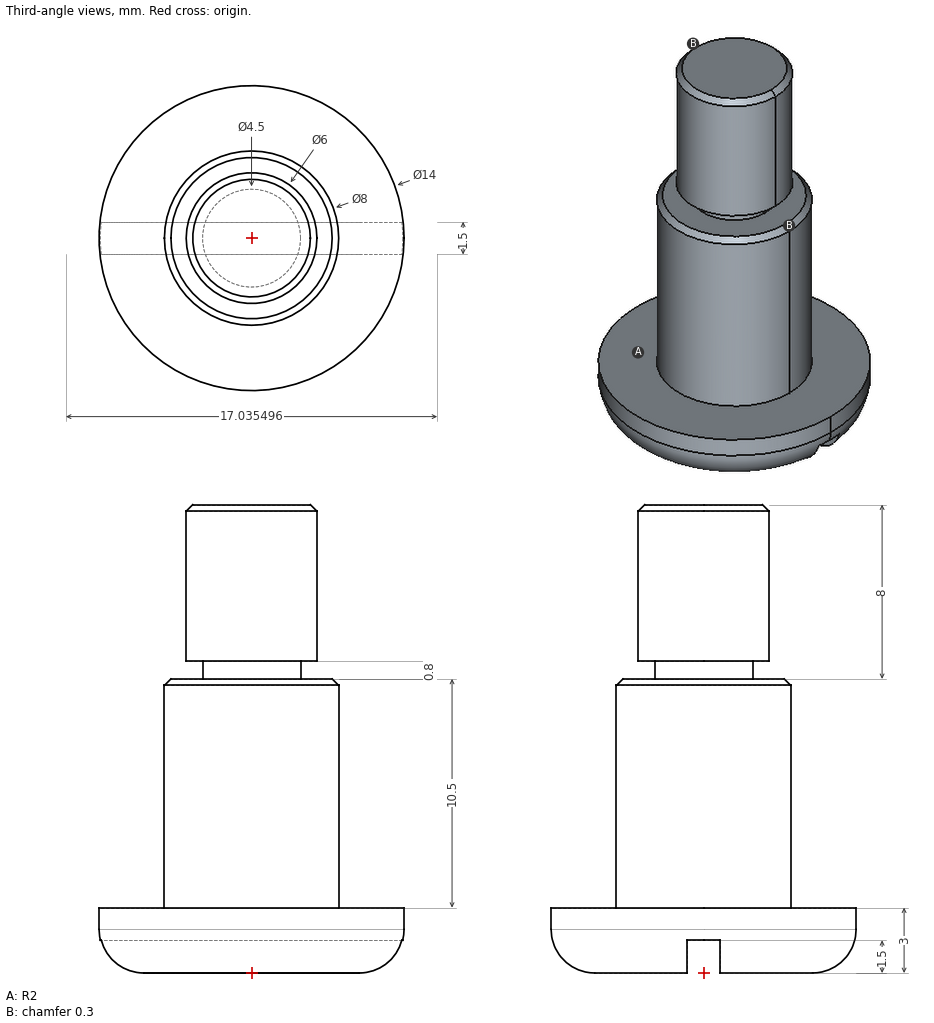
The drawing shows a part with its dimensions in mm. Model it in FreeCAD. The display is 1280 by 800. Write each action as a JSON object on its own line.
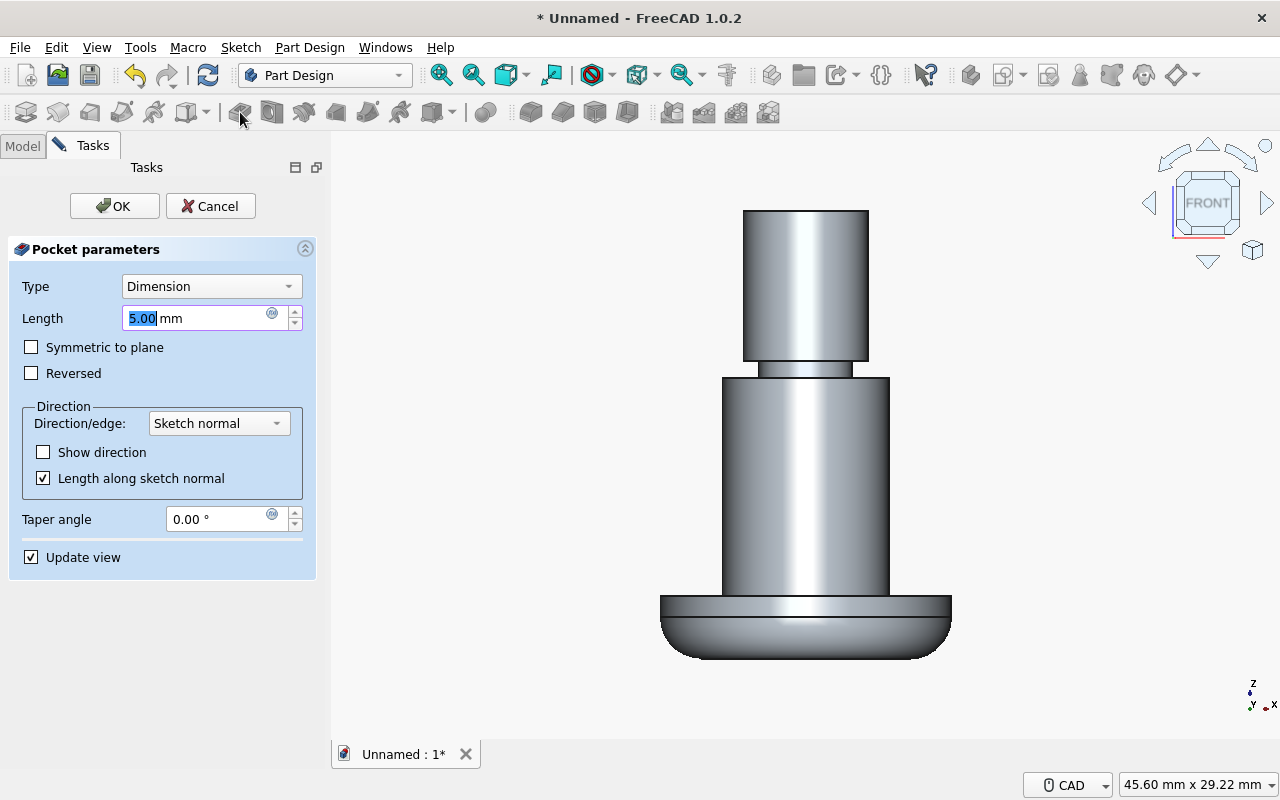
{"action": "type", "text": "1.5"}
{"action": "key", "text": "Tab"}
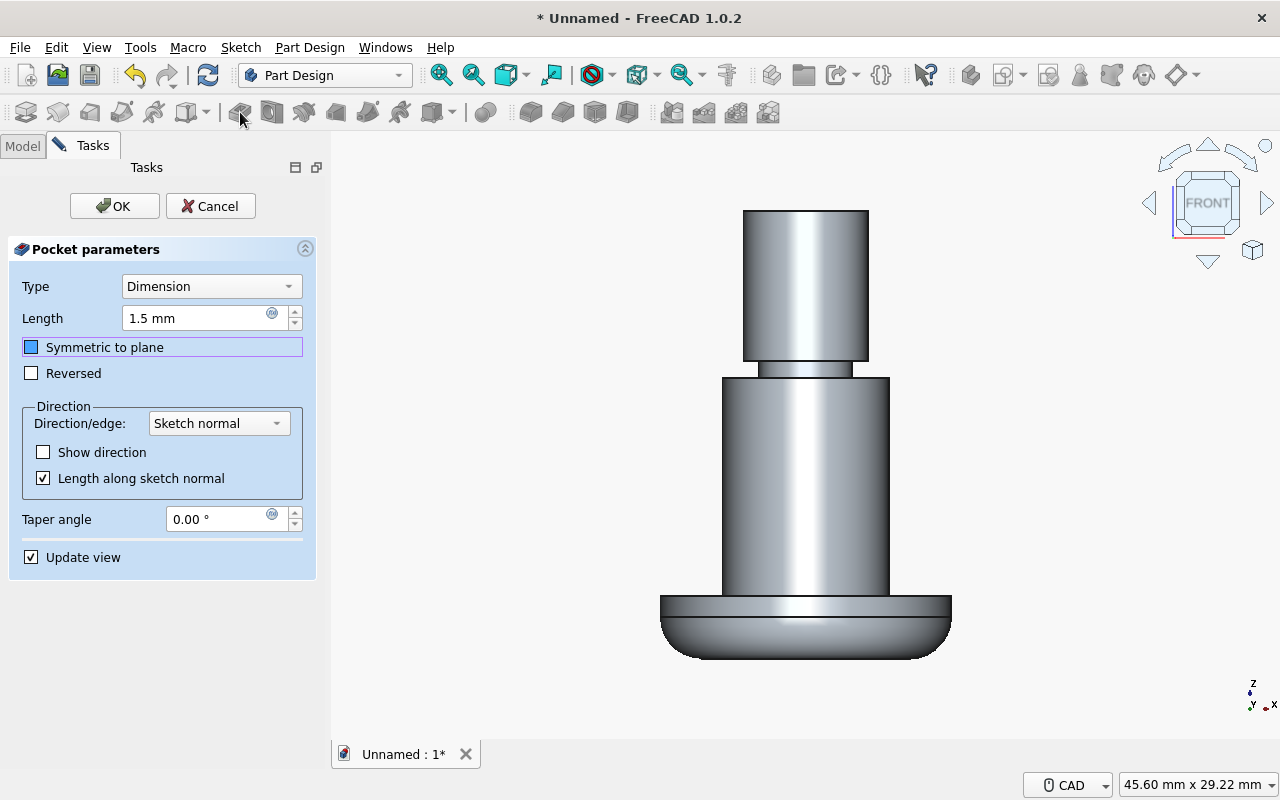
{"action": "left_click", "coordinate": [30, 373]}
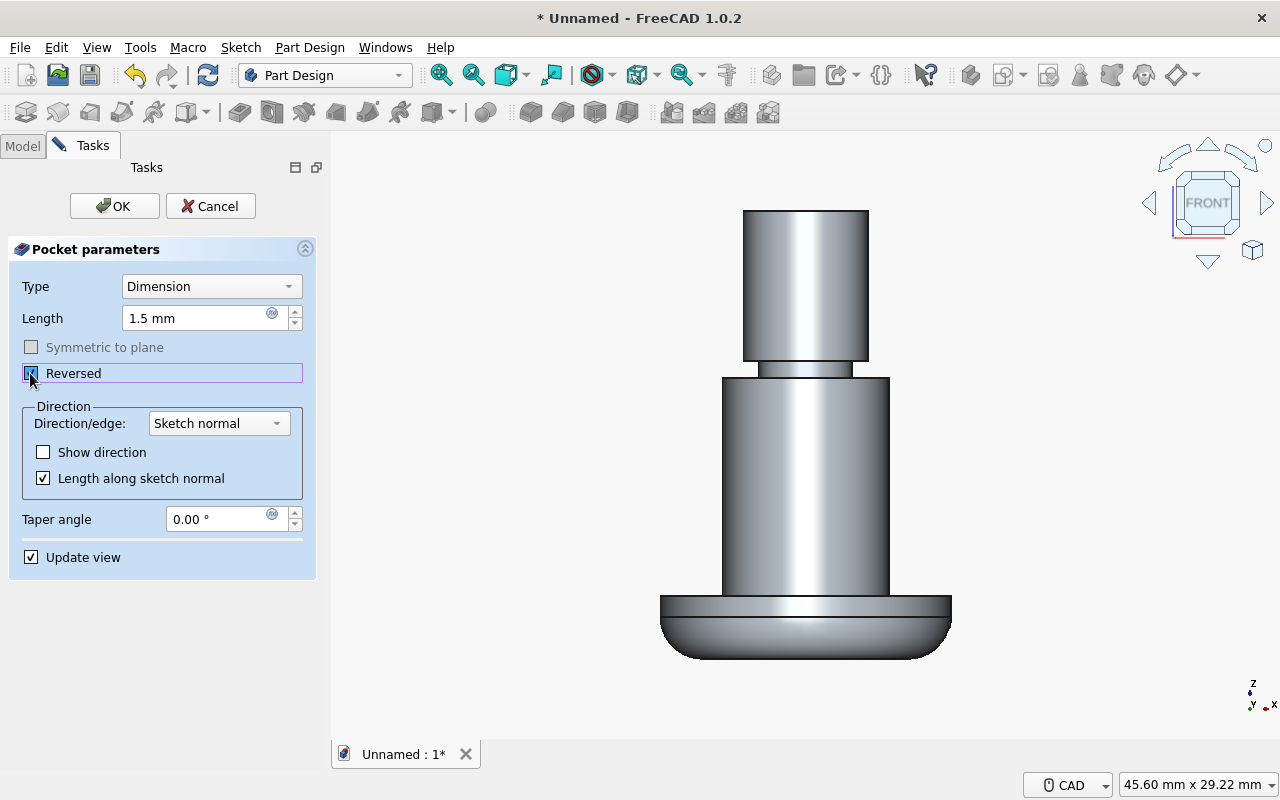
{"action": "left_click", "coordinate": [115, 206]}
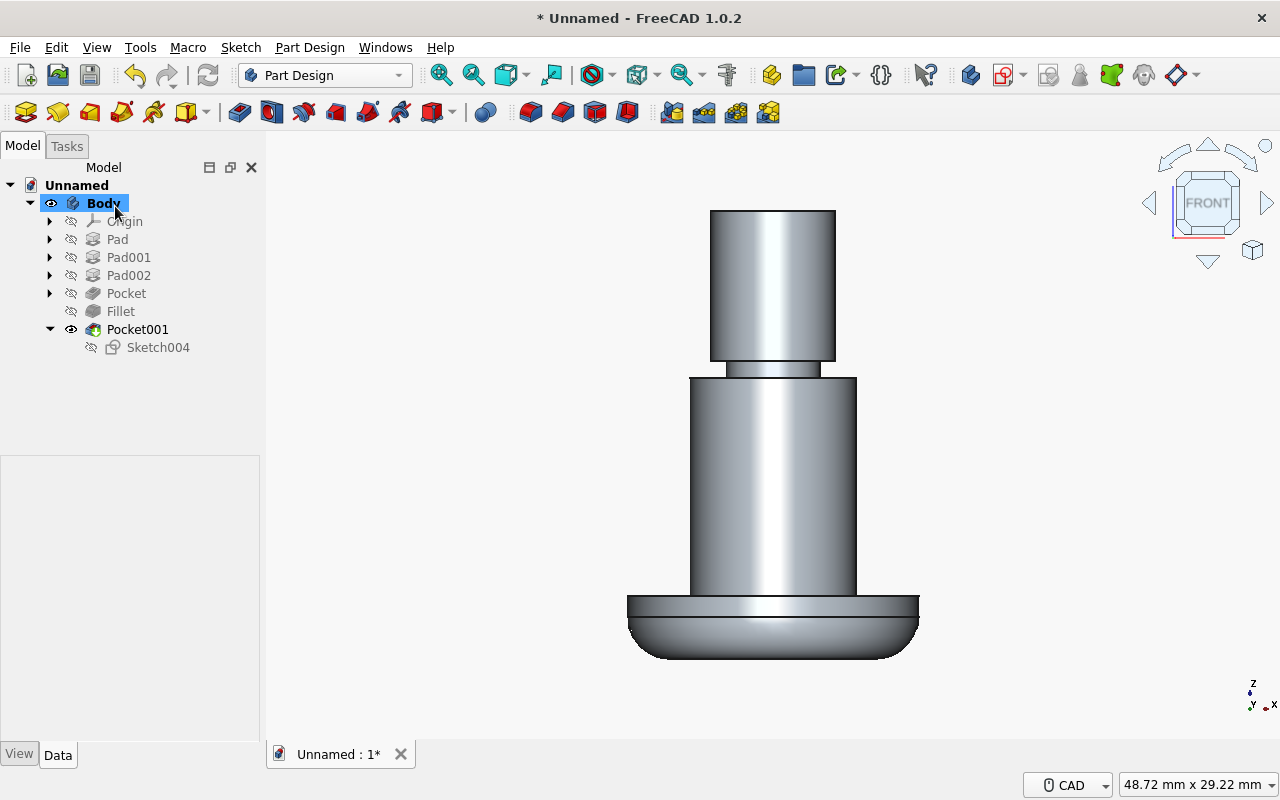
{"action": "left_click", "coordinate": [722, 210]}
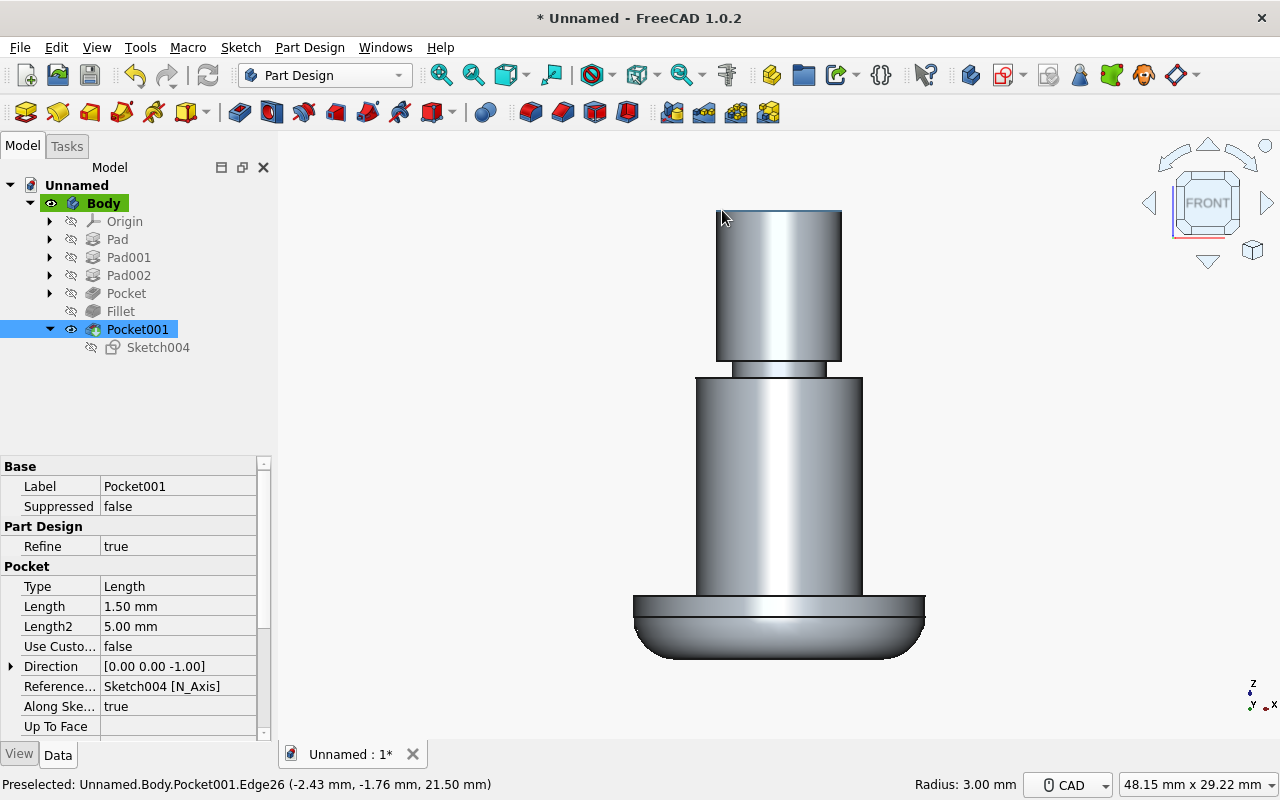
{"action": "left_click", "coordinate": [711, 377], "text": "ctrl"}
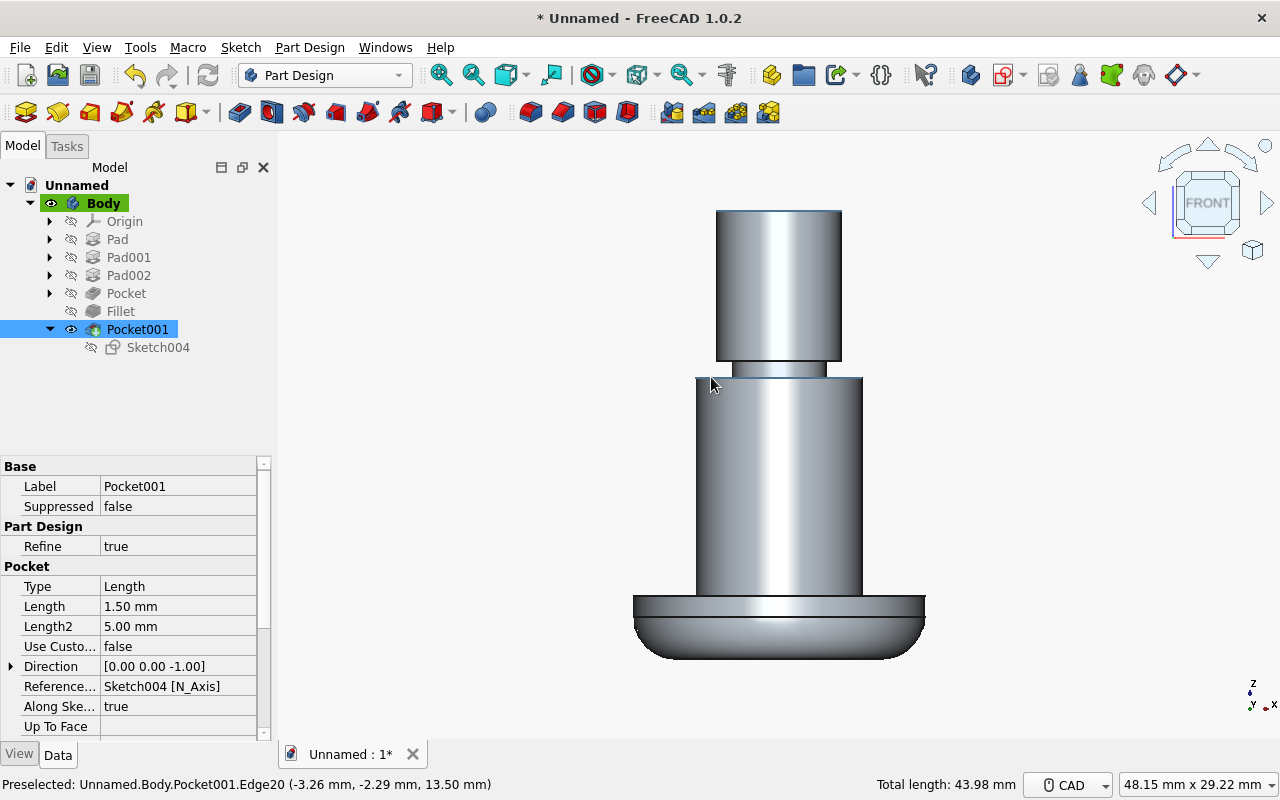
{"action": "left_click", "coordinate": [564, 112]}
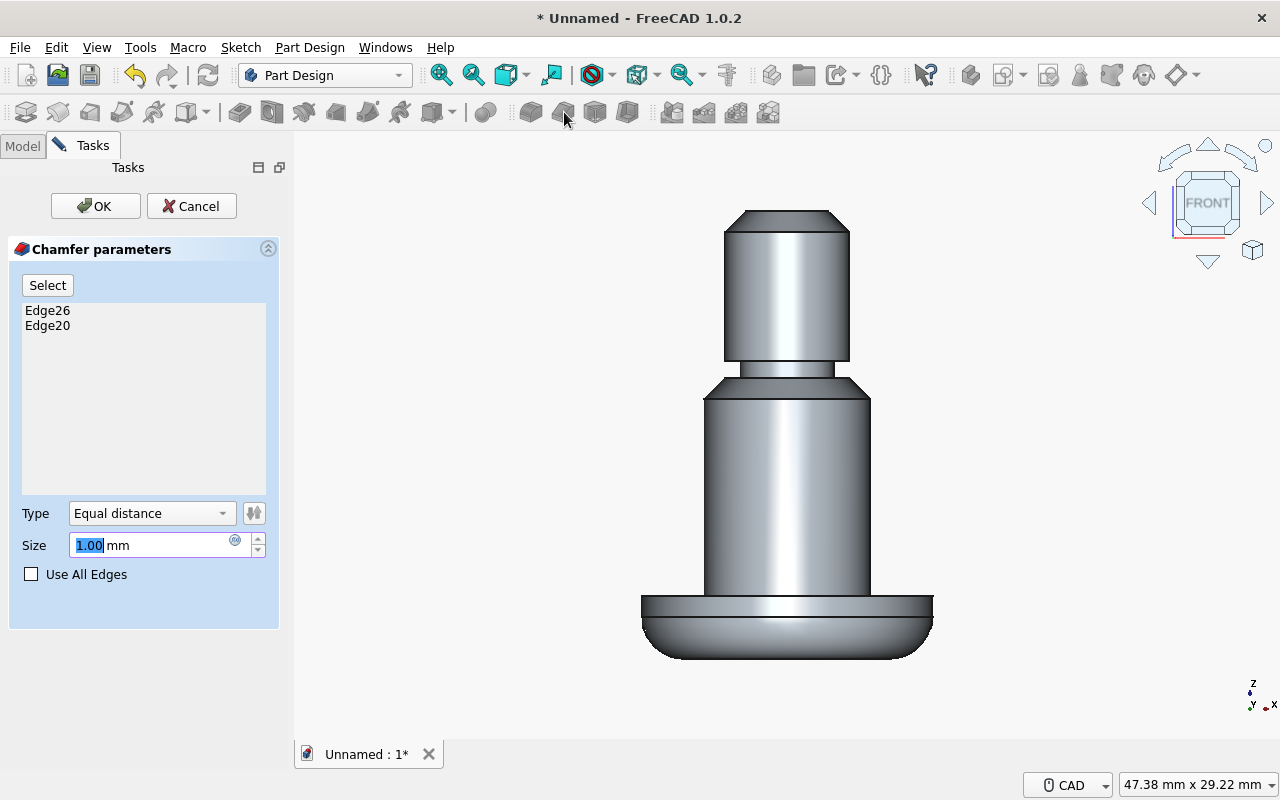
{"action": "type", "text": "0.3"}
{"action": "key", "text": "Tab"}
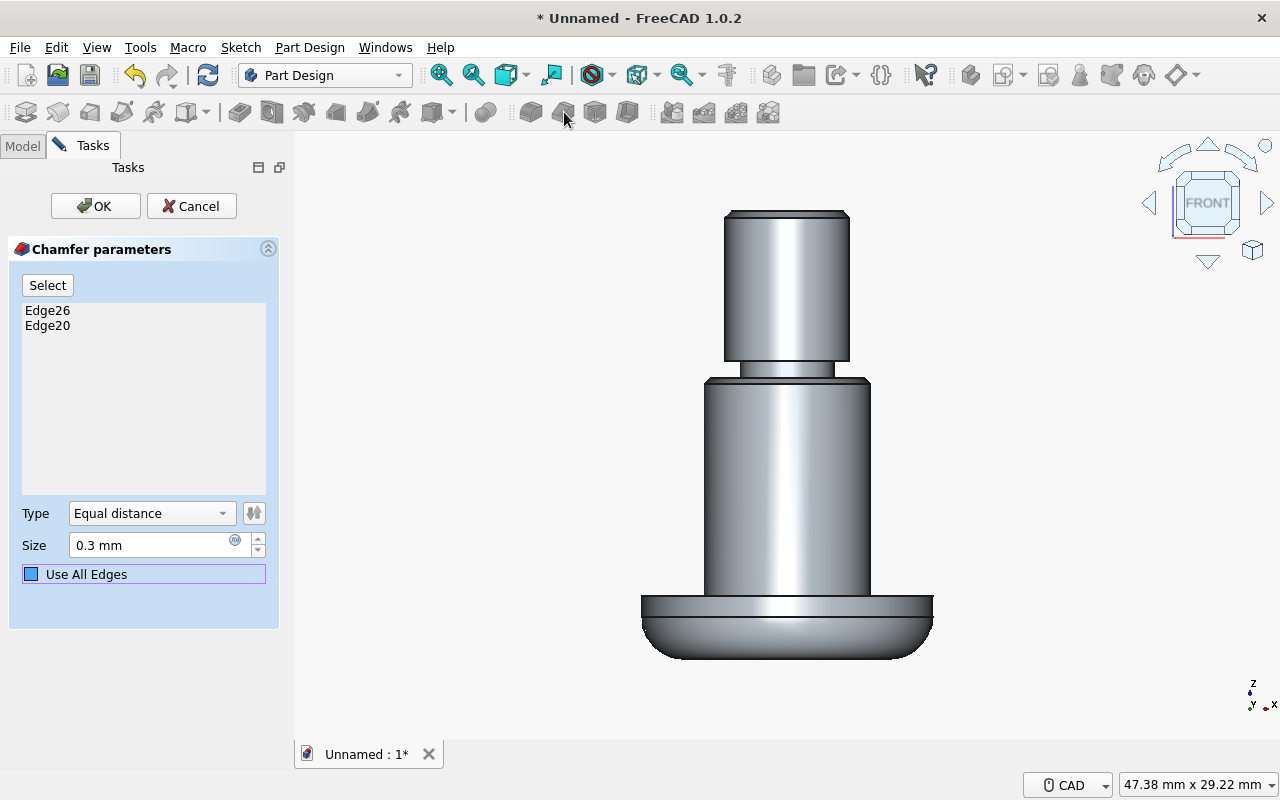
{"action": "left_click", "coordinate": [96, 206]}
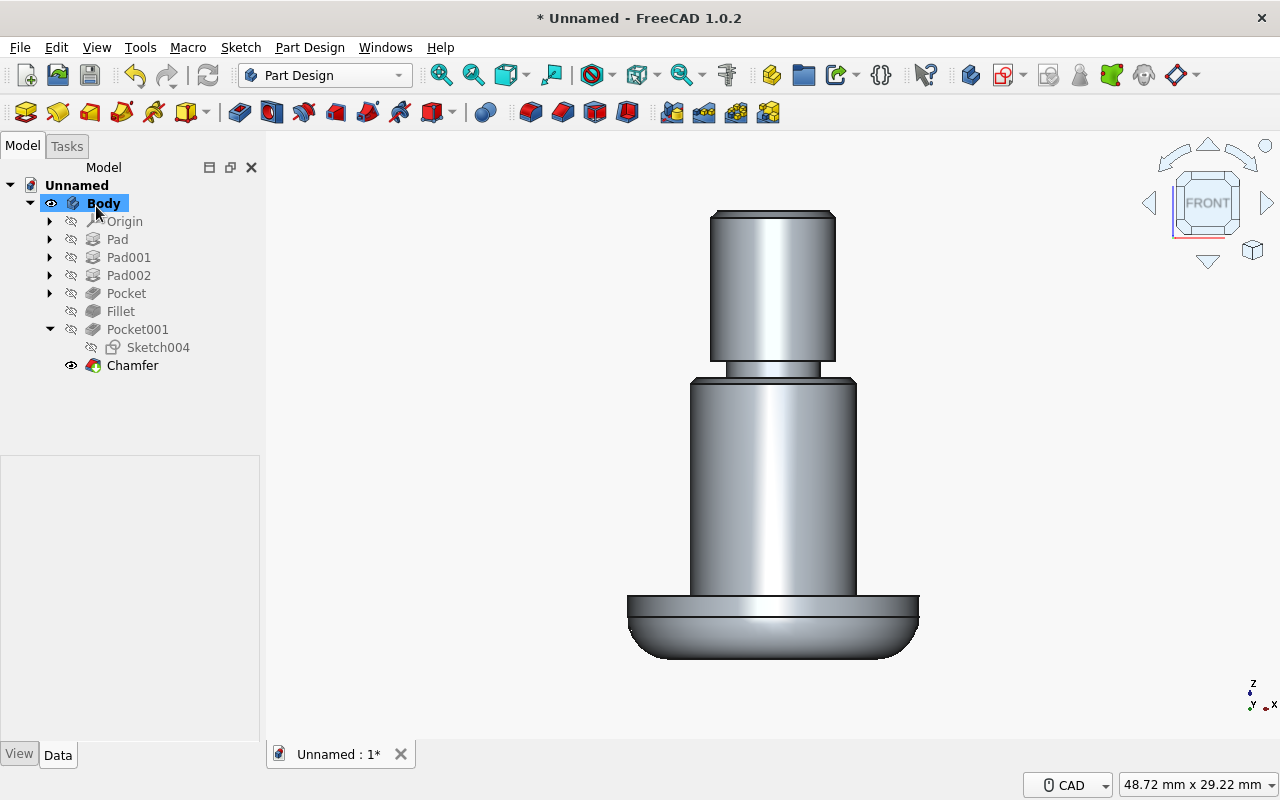
{"action": "key", "text": "0"}